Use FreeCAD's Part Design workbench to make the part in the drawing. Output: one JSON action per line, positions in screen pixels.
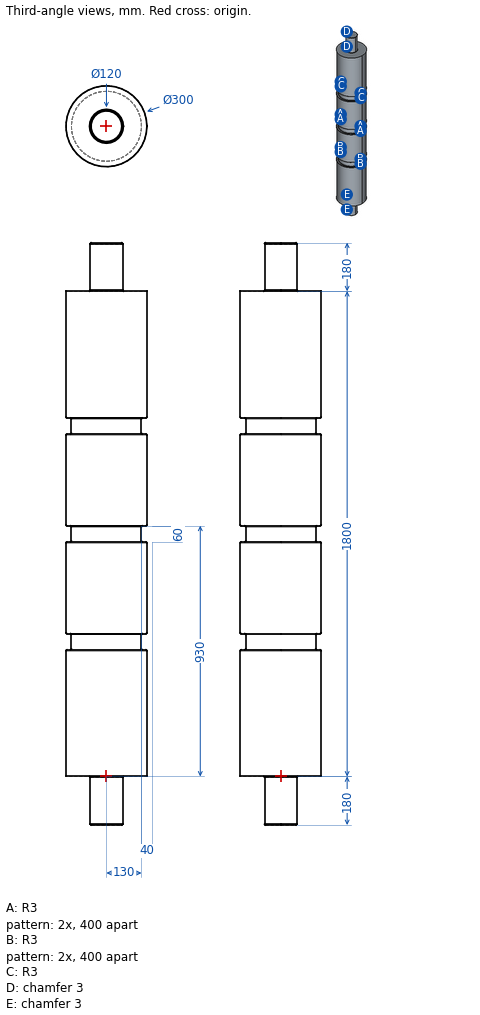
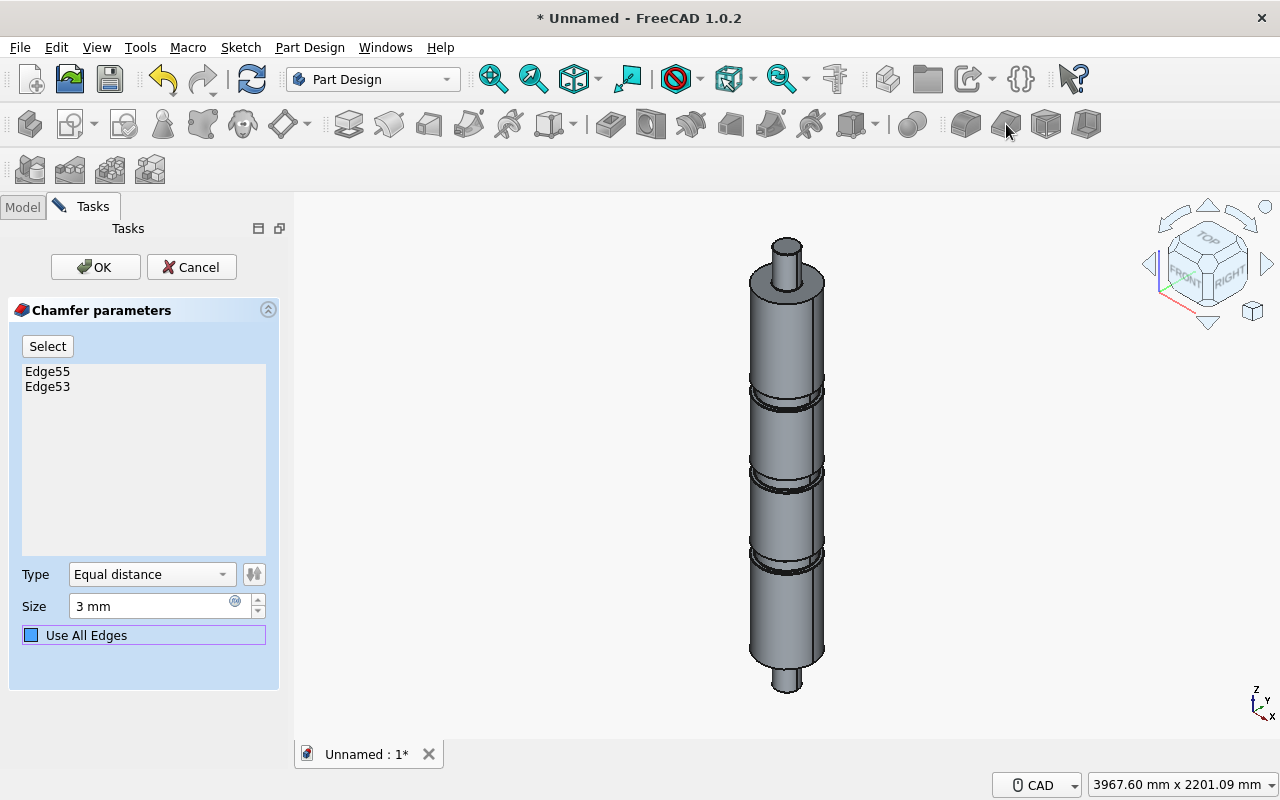
{"action": "left_click", "coordinate": [96, 267]}